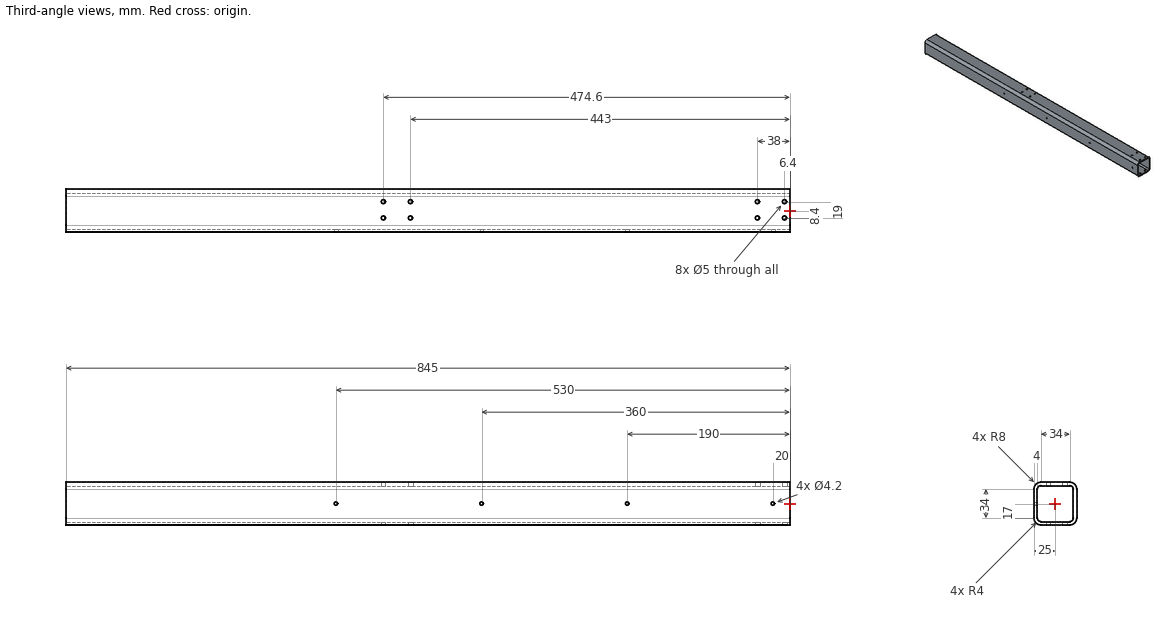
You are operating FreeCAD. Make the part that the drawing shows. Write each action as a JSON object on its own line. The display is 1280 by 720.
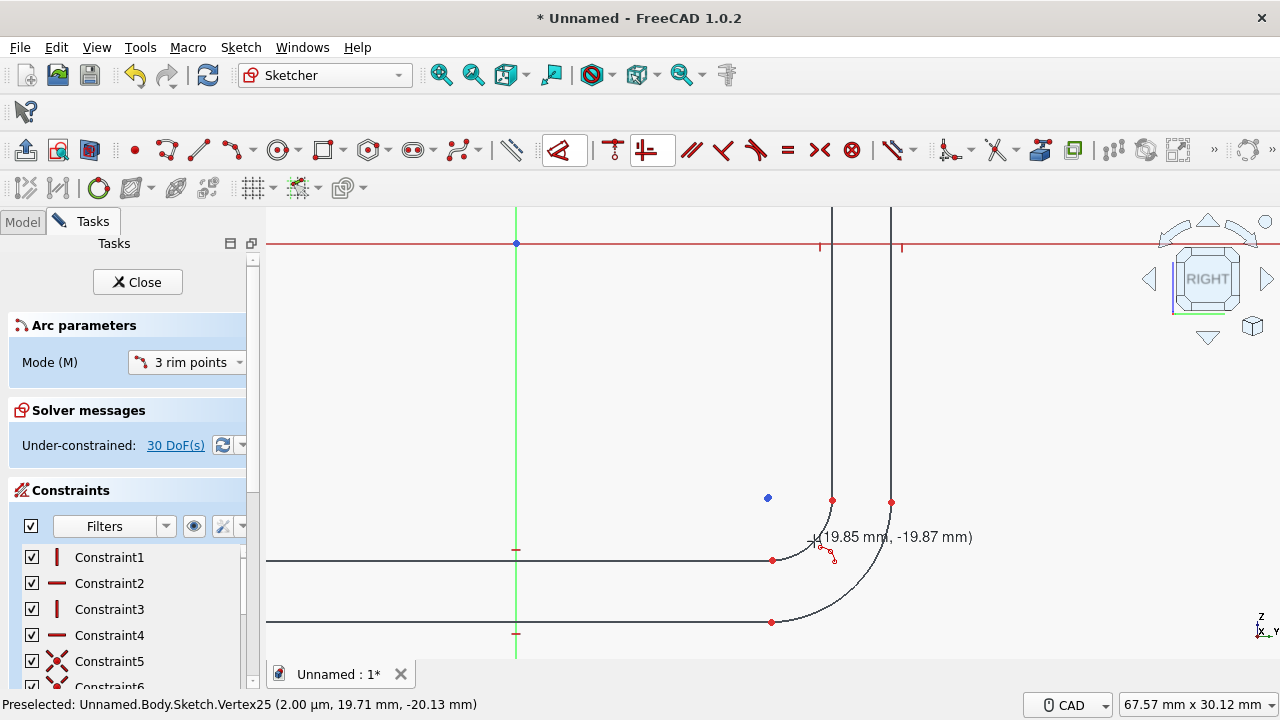
{"action": "scroll", "coordinate": [814, 543], "scroll_direction": "down", "scroll_amount": 5}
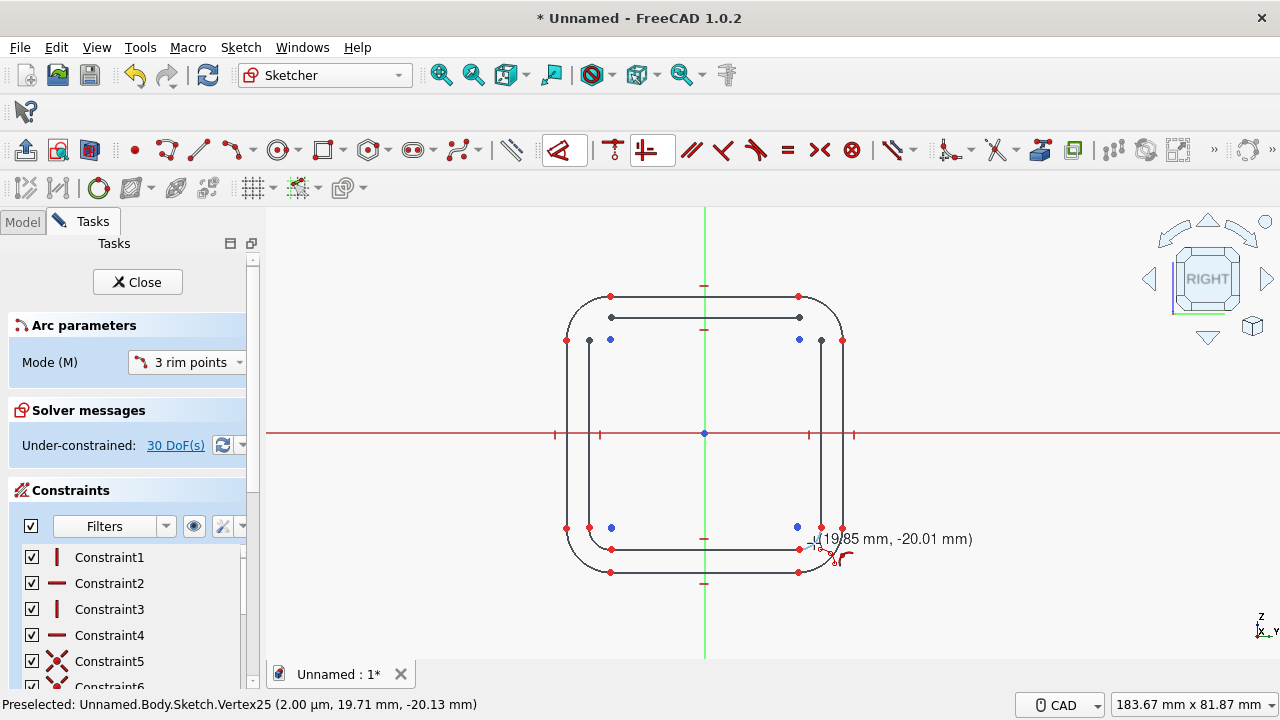
{"action": "left_click", "coordinate": [821, 341]}
{"action": "left_click", "coordinate": [799, 318]}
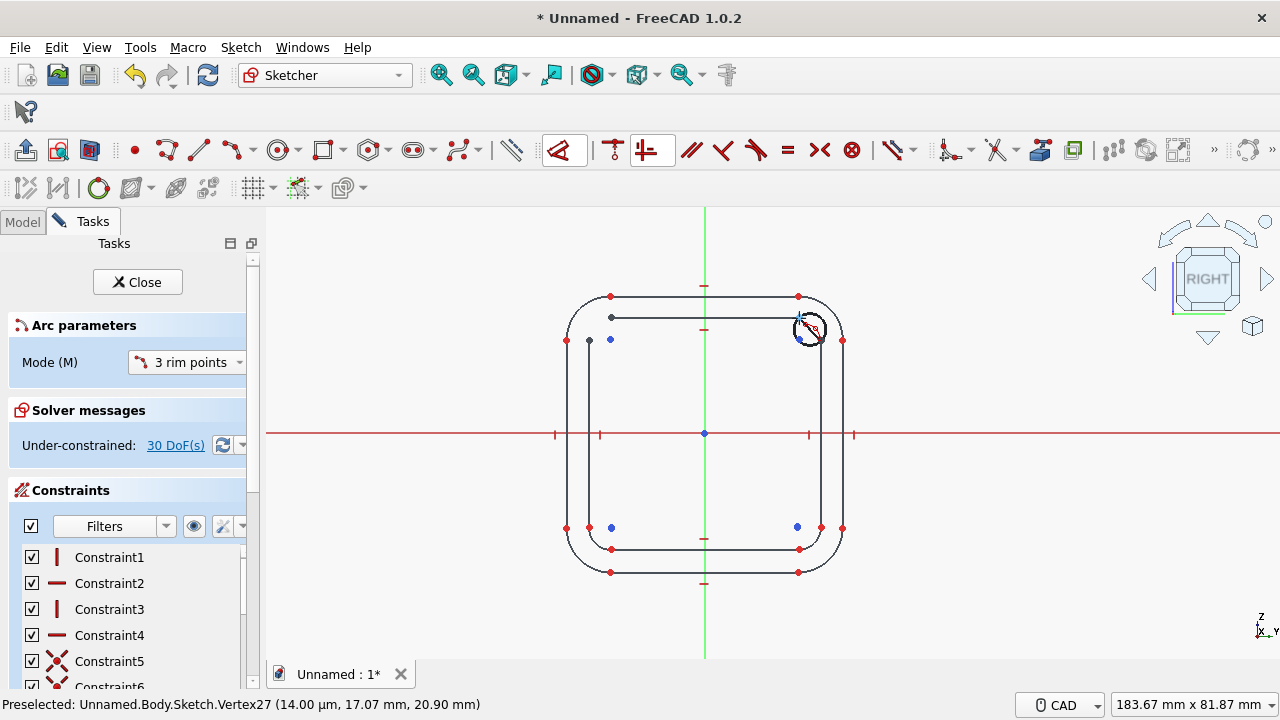
{"action": "scroll", "coordinate": [814, 324], "scroll_direction": "up", "scroll_amount": 5}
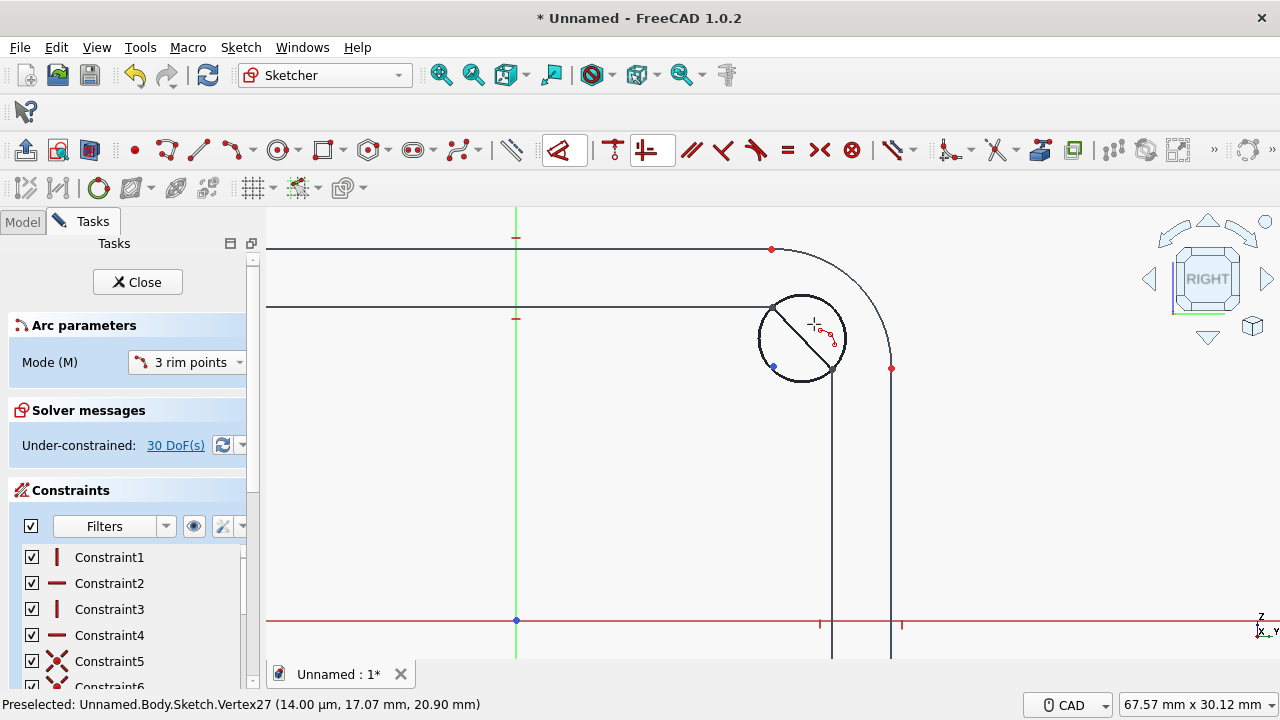
{"action": "left_click", "coordinate": [814, 323]}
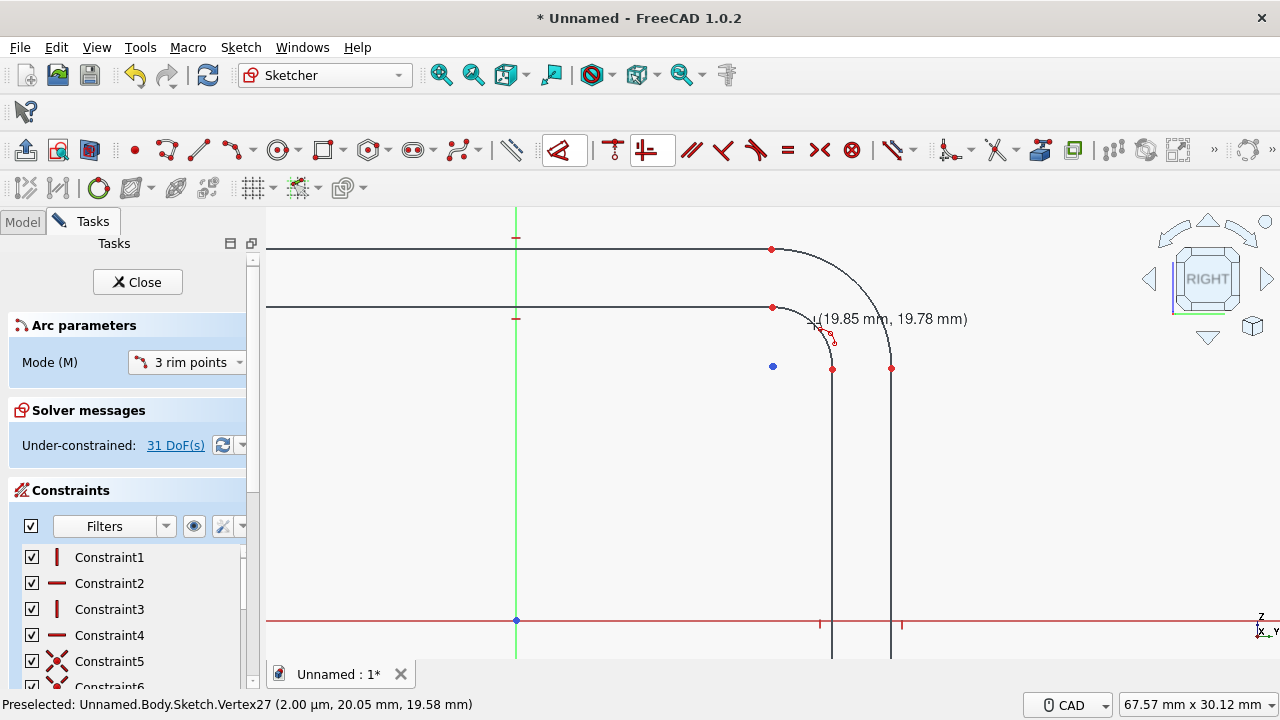
{"action": "scroll", "coordinate": [814, 324], "scroll_direction": "down", "scroll_amount": 5}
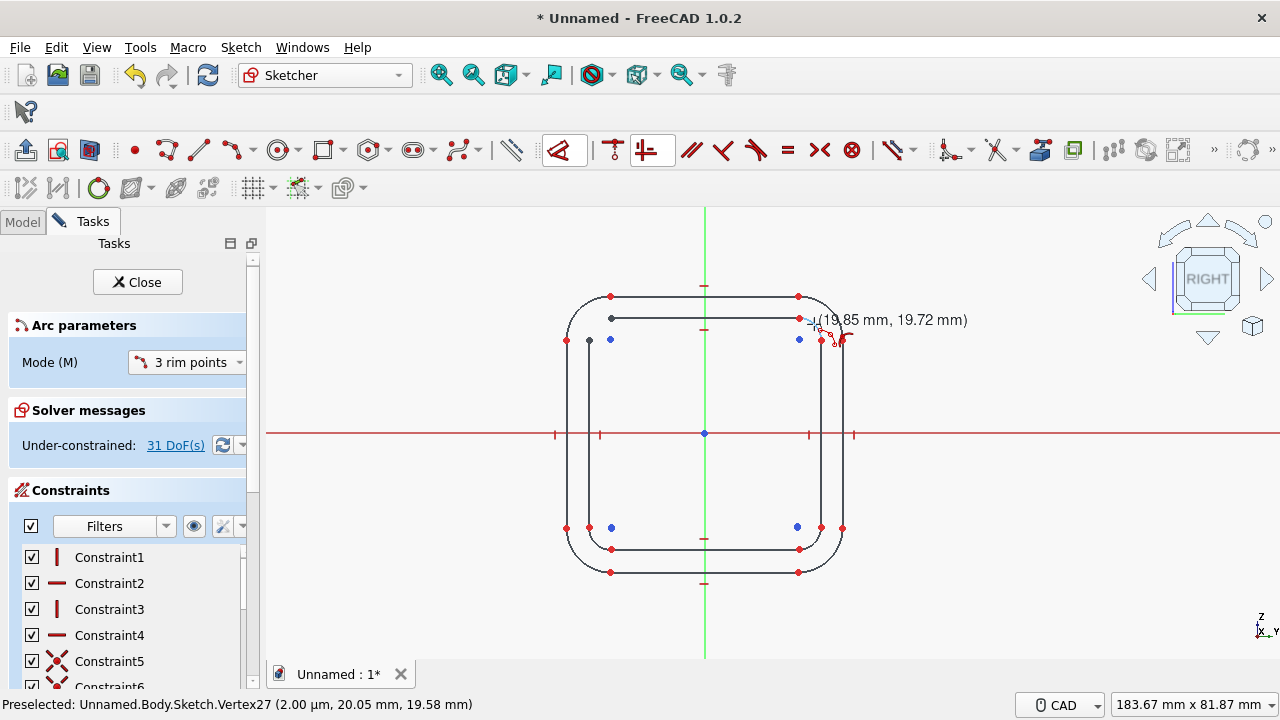
{"action": "left_click", "coordinate": [611, 318]}
{"action": "left_click", "coordinate": [589, 341]}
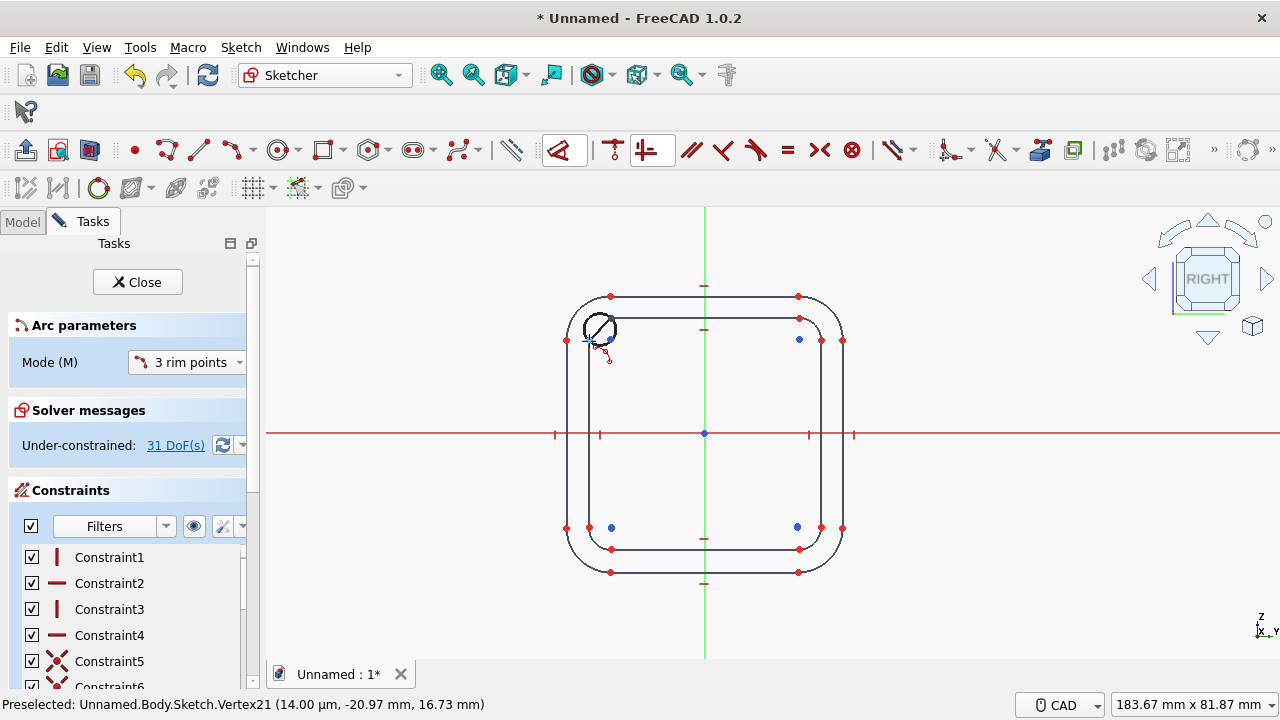
{"action": "scroll", "coordinate": [595, 324], "scroll_direction": "up", "scroll_amount": 5}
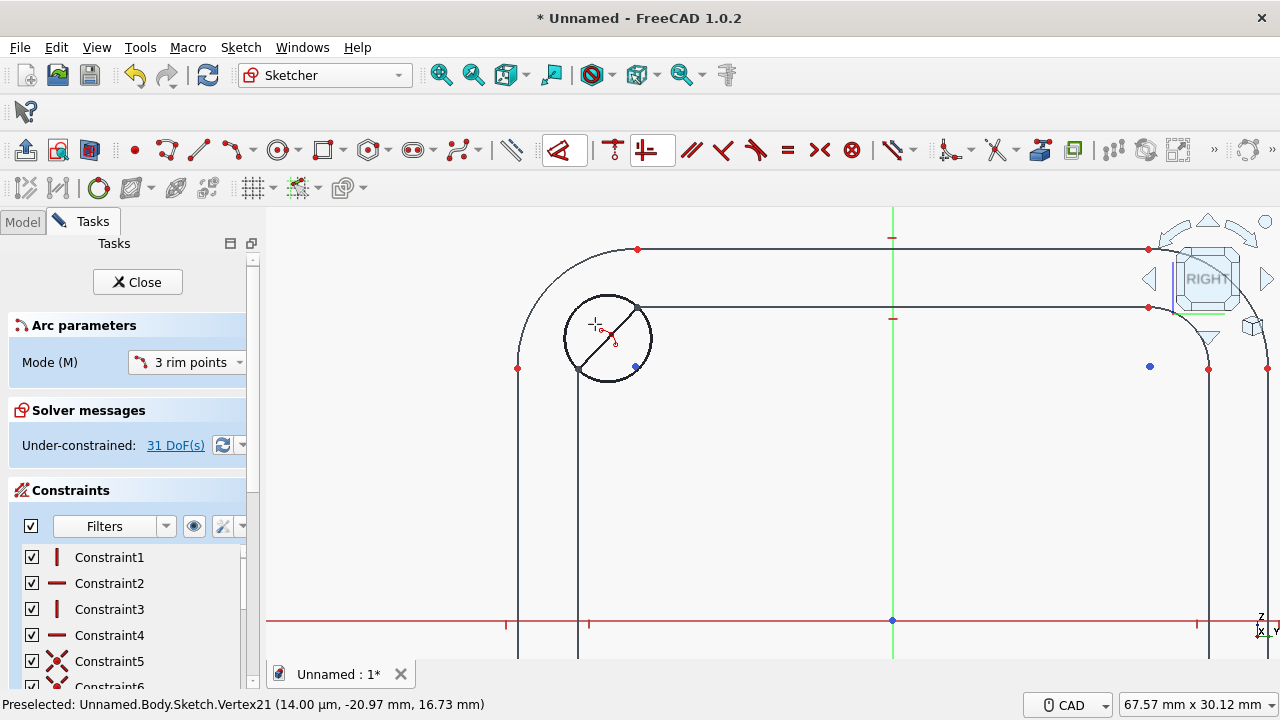
{"action": "left_click", "coordinate": [595, 323]}
{"action": "key", "text": "Escape"}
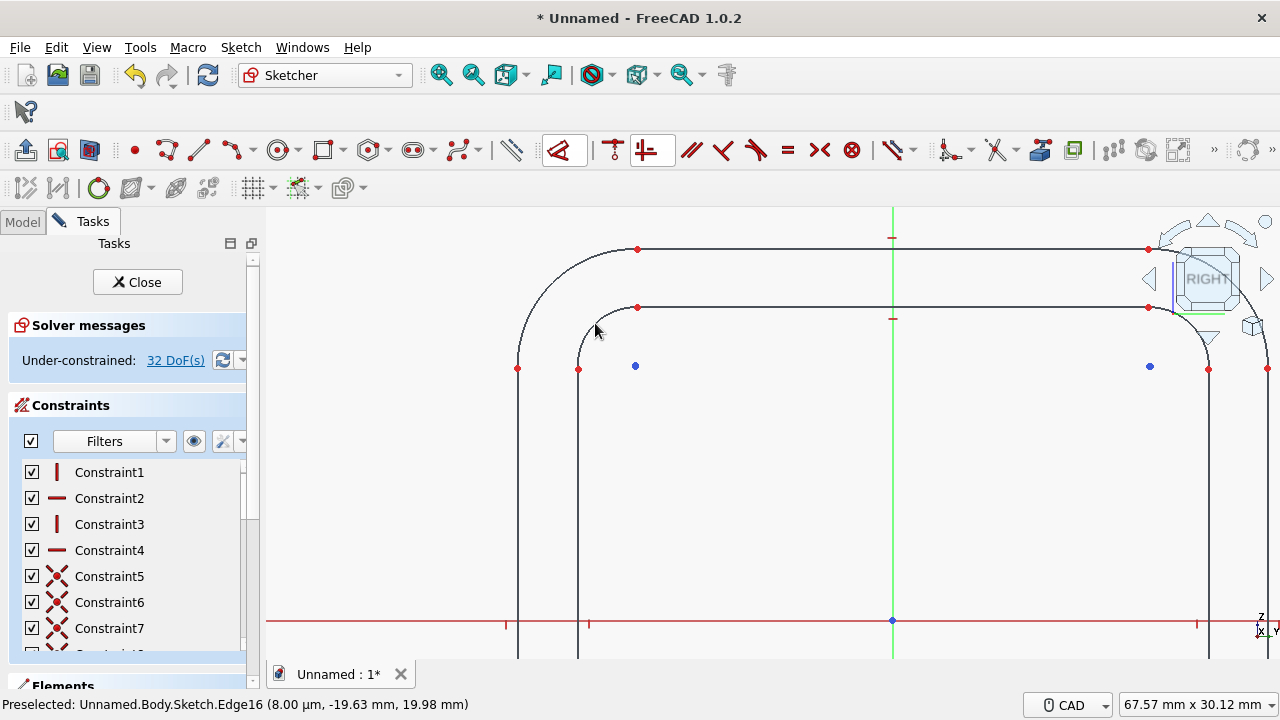
{"action": "left_click", "coordinate": [518, 522]}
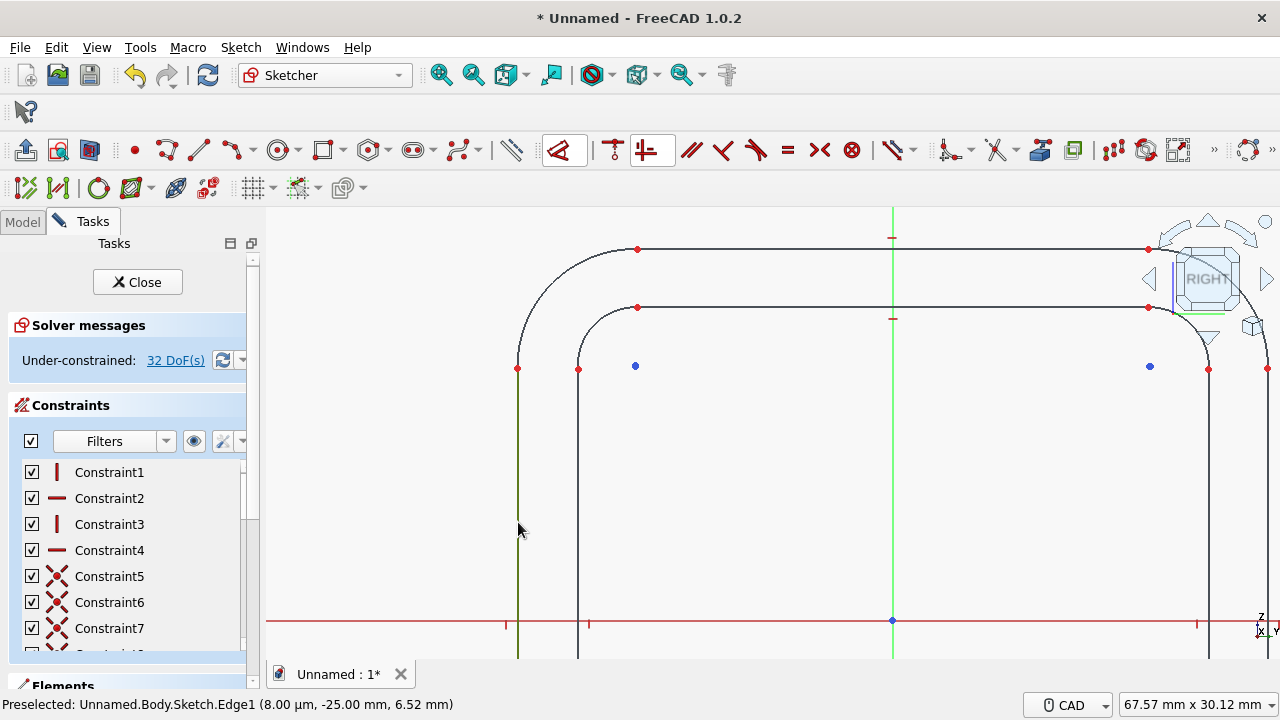
{"action": "left_click", "coordinate": [582, 262]}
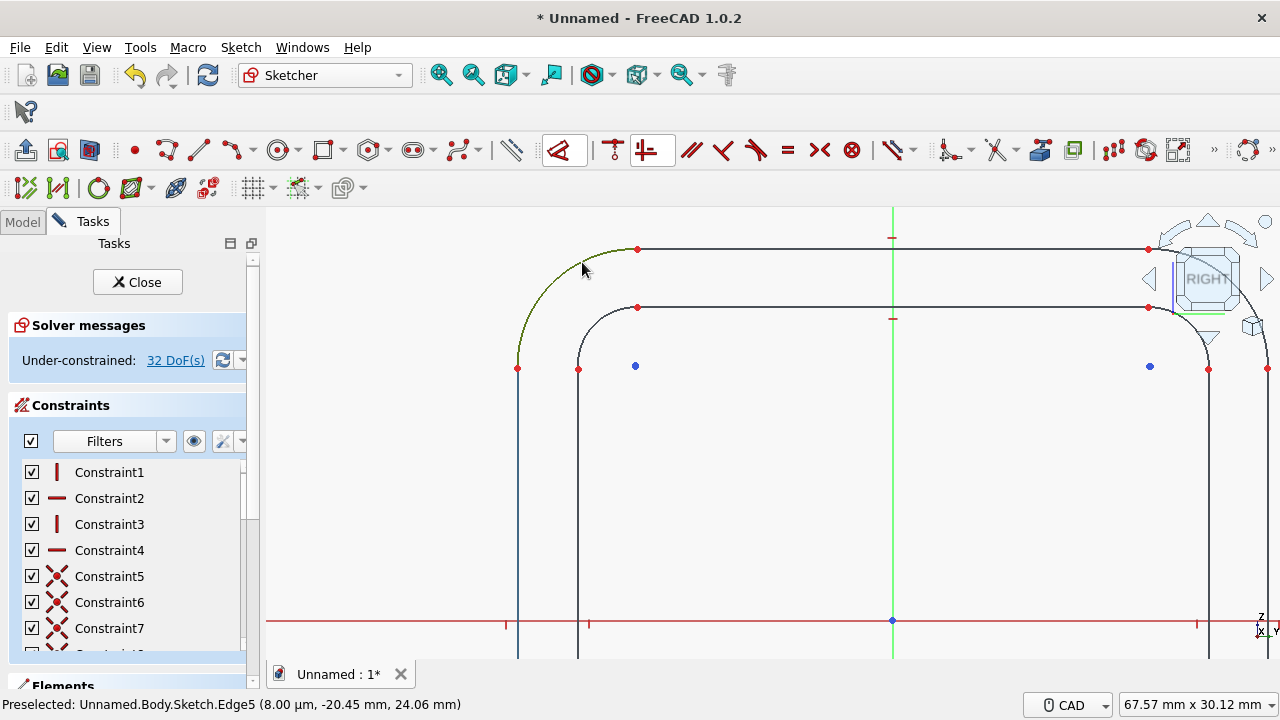
{"action": "left_click", "coordinate": [756, 150]}